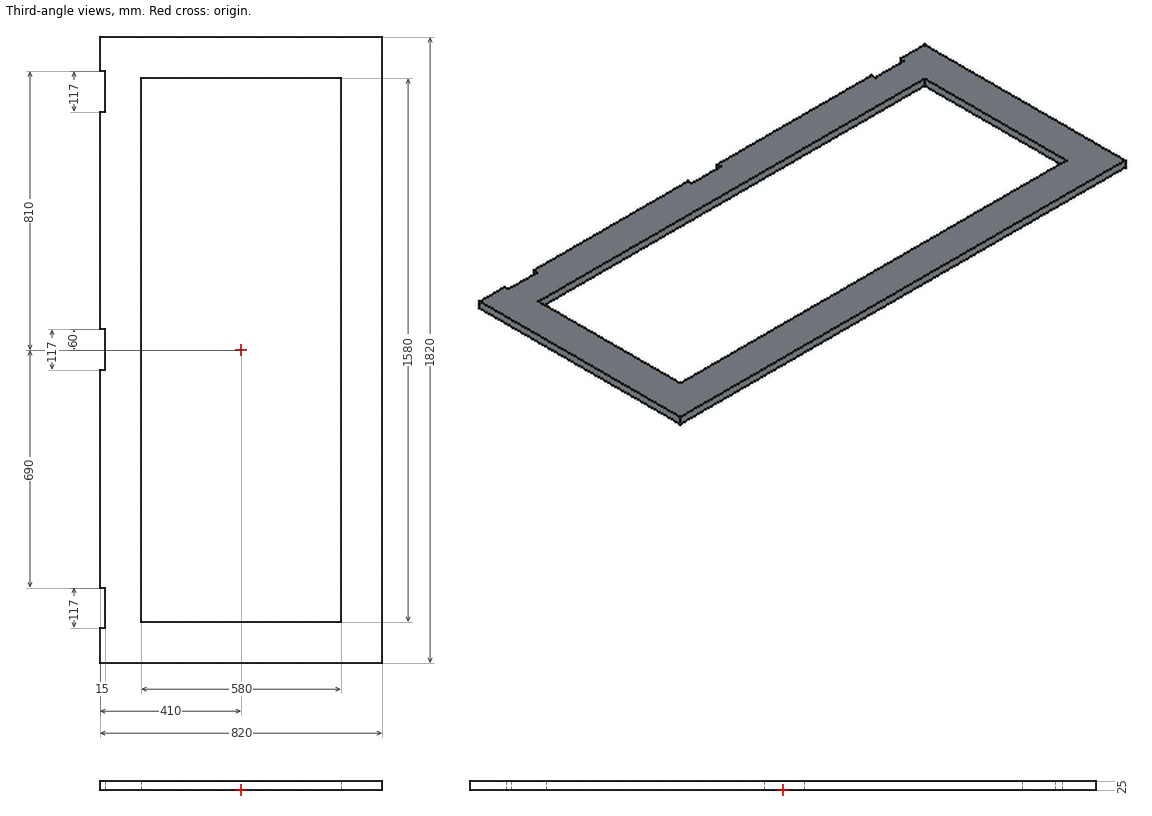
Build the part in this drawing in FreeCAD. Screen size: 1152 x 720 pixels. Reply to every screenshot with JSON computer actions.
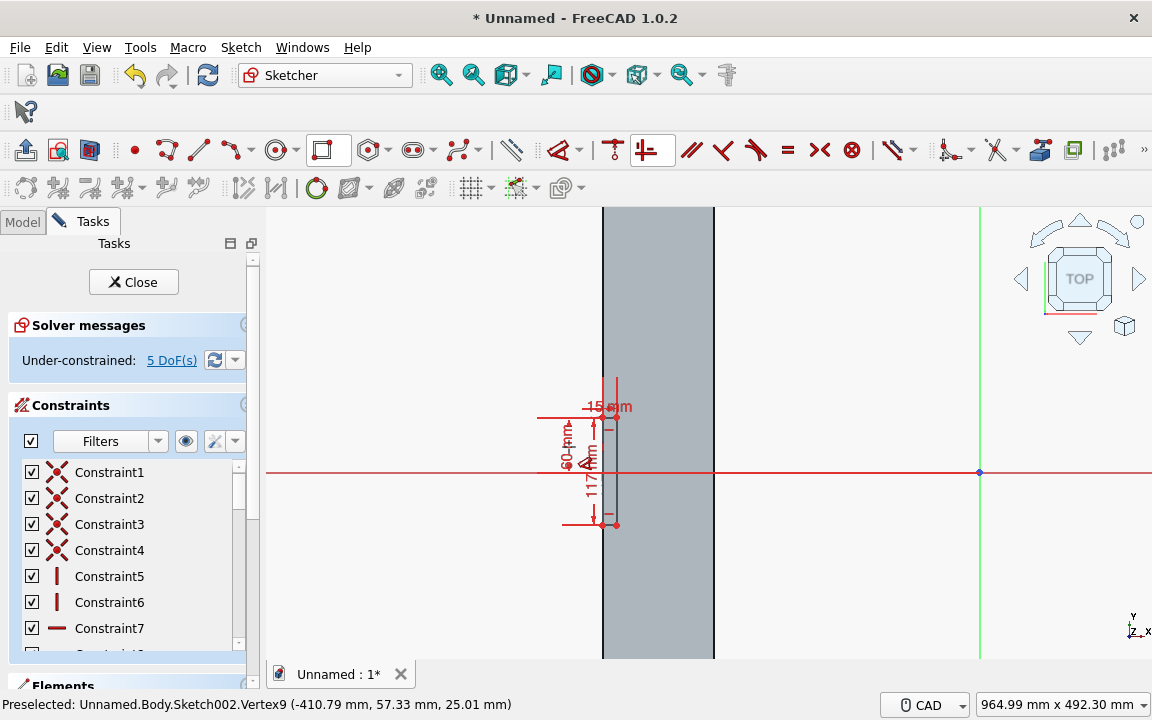
{"action": "scroll", "coordinate": [602, 423], "scroll_direction": "down", "scroll_amount": 8}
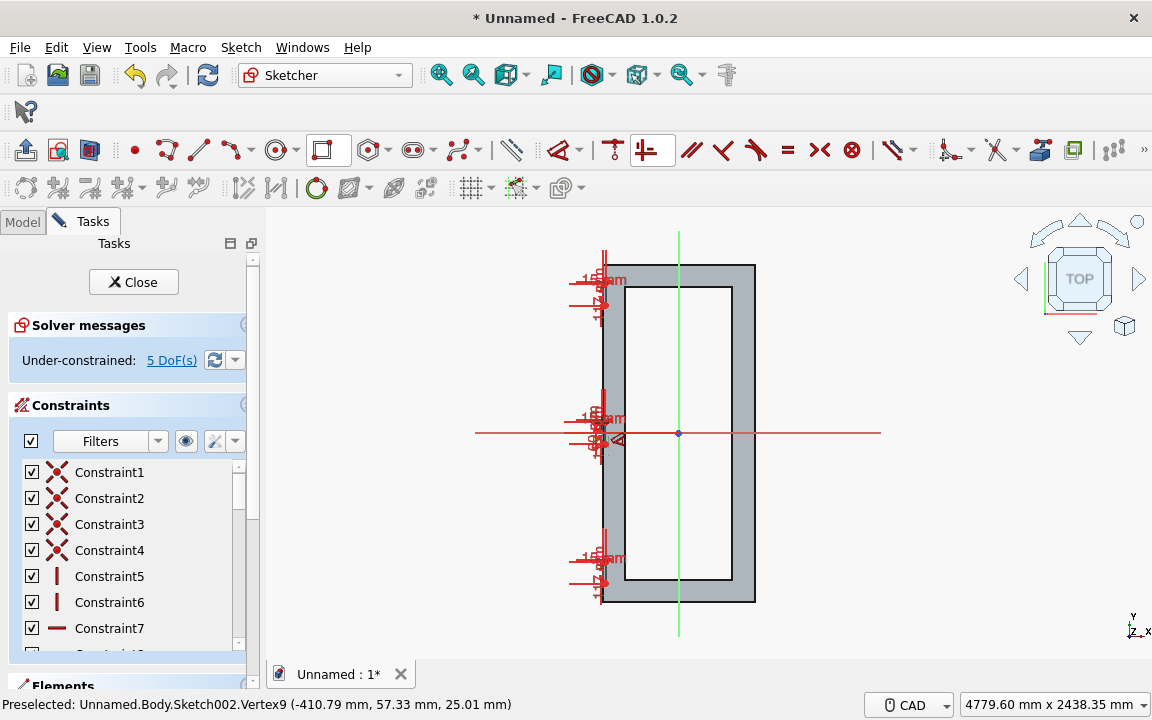
{"action": "scroll", "coordinate": [603, 562], "scroll_direction": "up", "scroll_amount": 8}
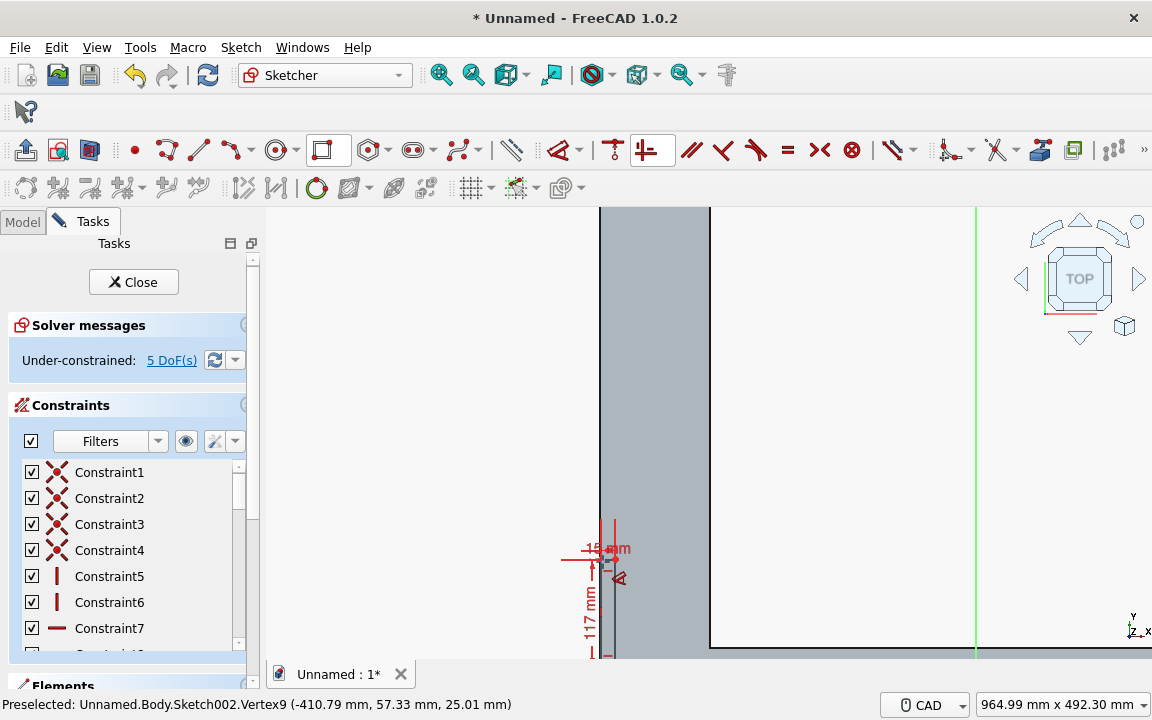
{"action": "left_click", "coordinate": [601, 560]}
{"action": "left_click", "coordinate": [789, 594]}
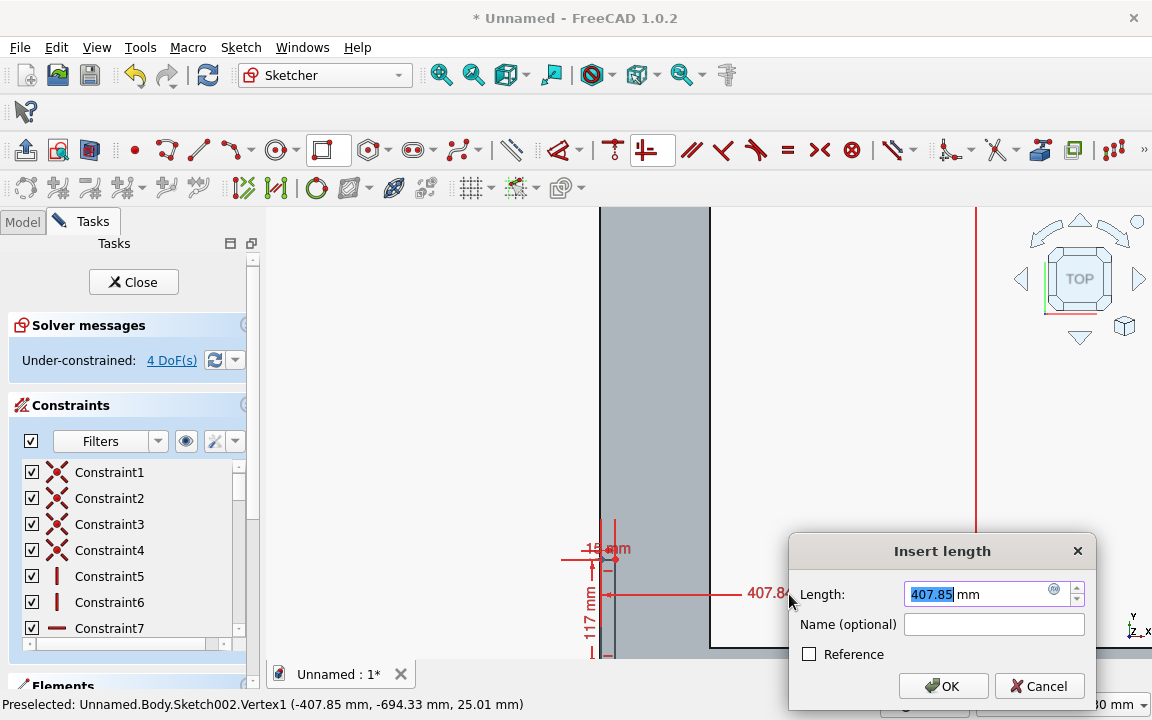
{"action": "type", "text": "410"}
{"action": "key", "text": "Return"}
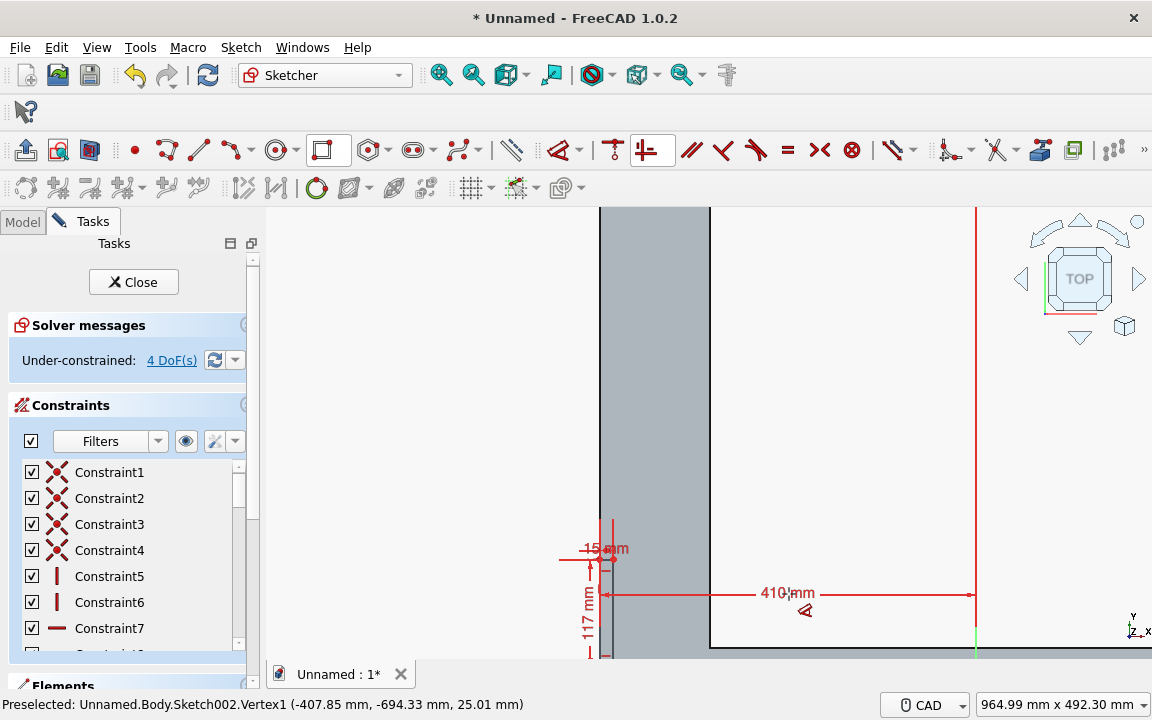
{"action": "left_click", "coordinate": [600, 560]}
{"action": "left_click", "coordinate": [566, 397]}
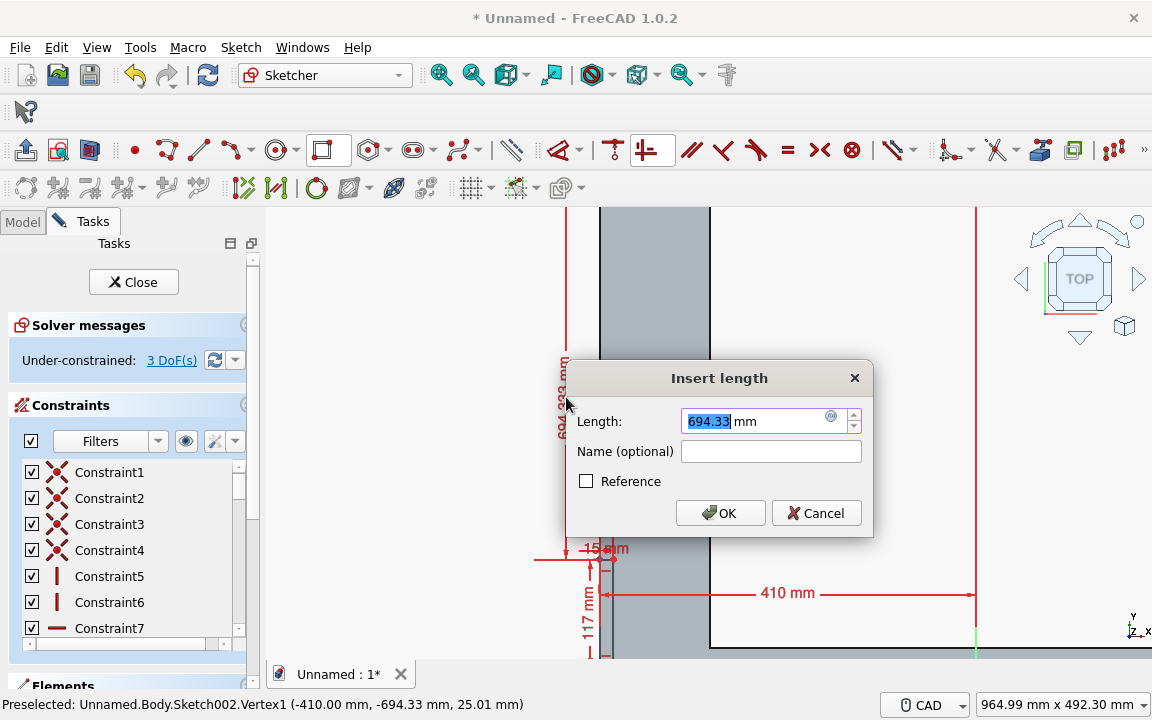
{"action": "type", "text": "690"}
{"action": "key", "text": "Return"}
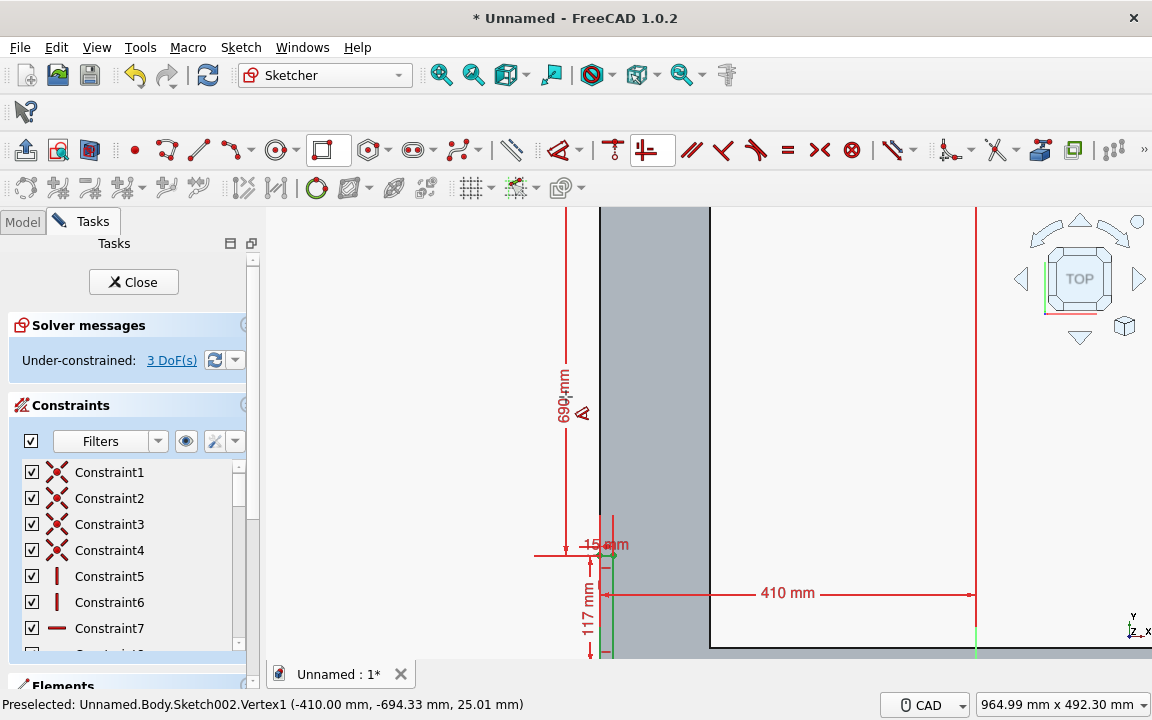
{"action": "scroll", "coordinate": [603, 563], "scroll_direction": "down", "scroll_amount": 8}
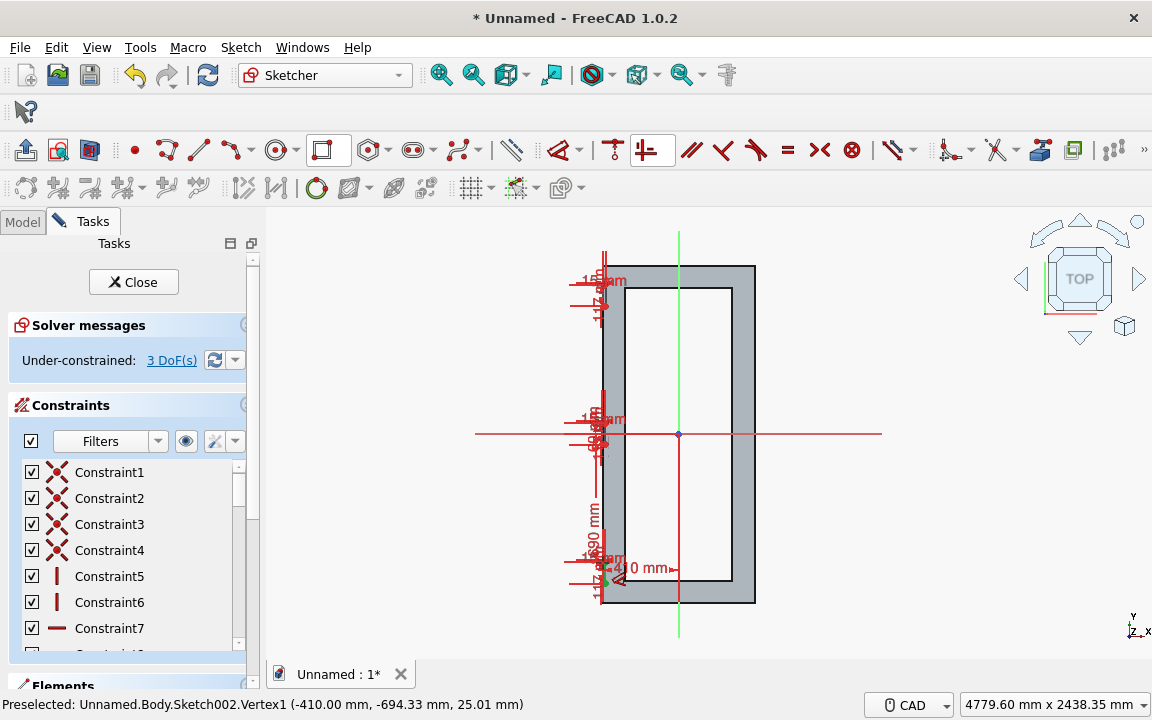
{"action": "scroll", "coordinate": [602, 423], "scroll_direction": "up", "scroll_amount": 8}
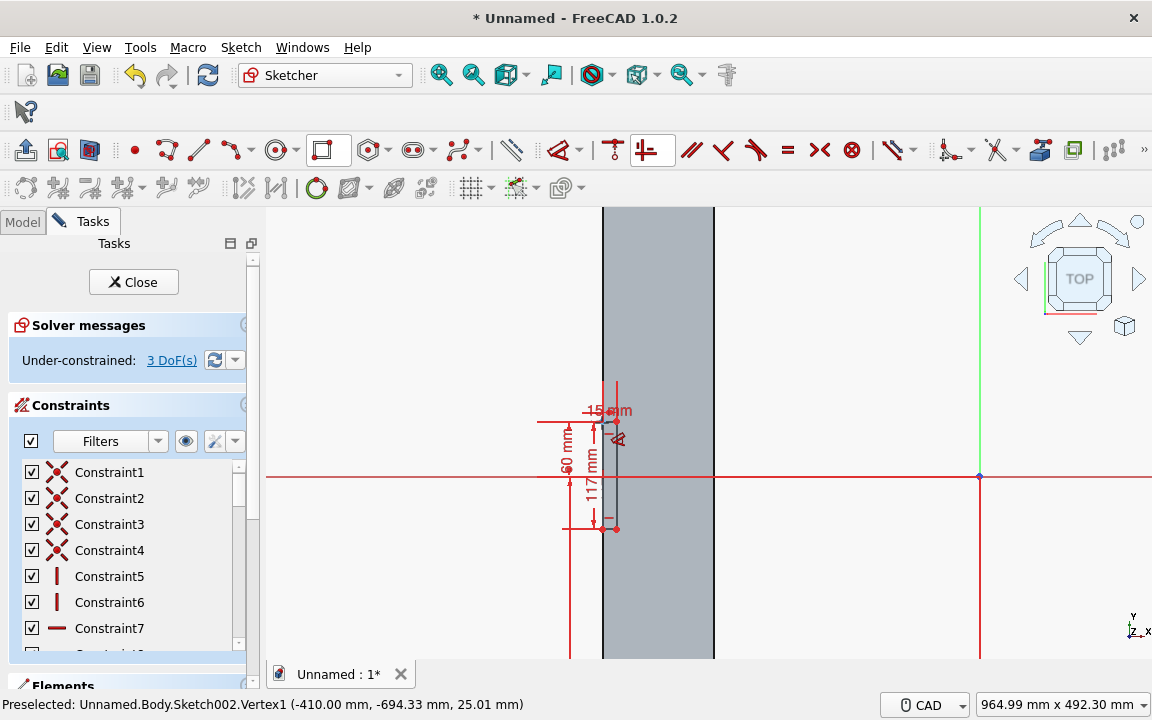
{"action": "left_click", "coordinate": [603, 422]}
{"action": "left_click", "coordinate": [791, 388]}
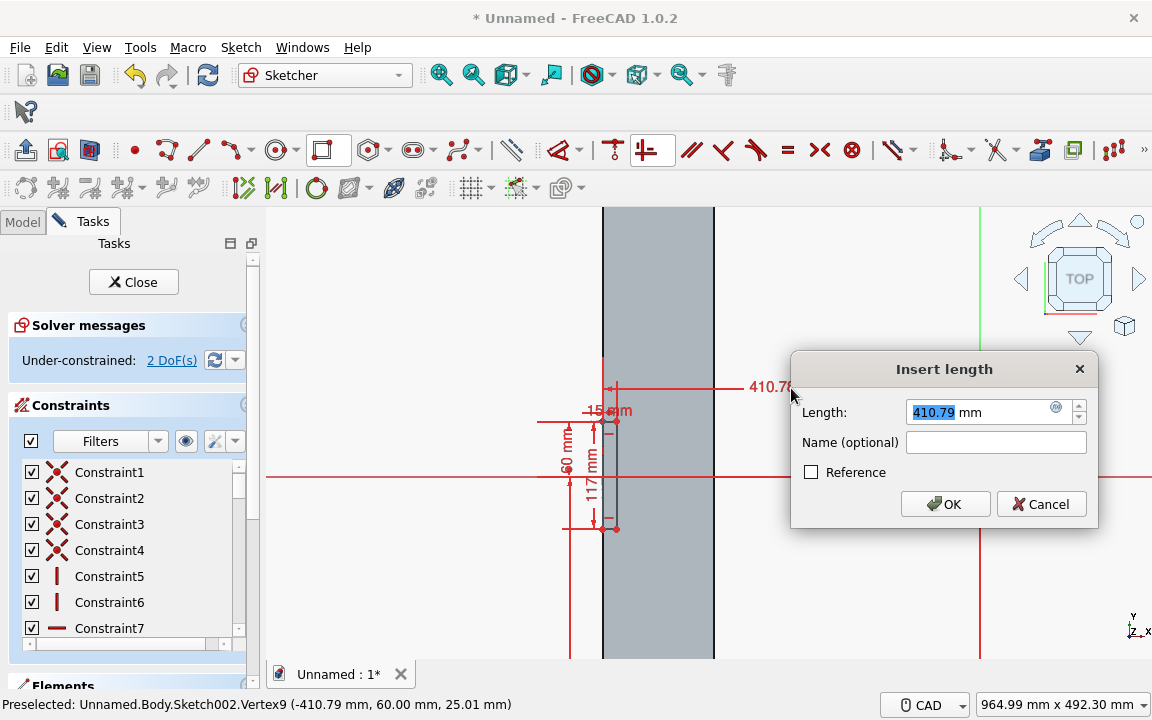
{"action": "type", "text": "410"}
{"action": "key", "text": "Return"}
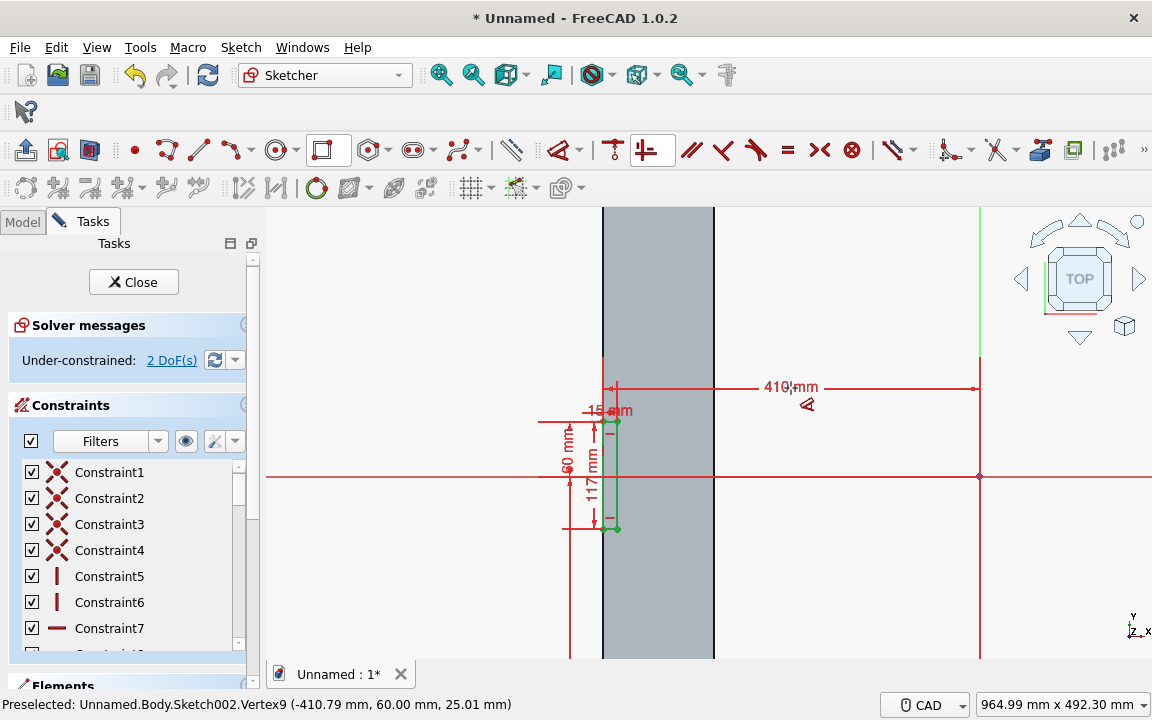
{"action": "scroll", "coordinate": [602, 422], "scroll_direction": "down", "scroll_amount": 8}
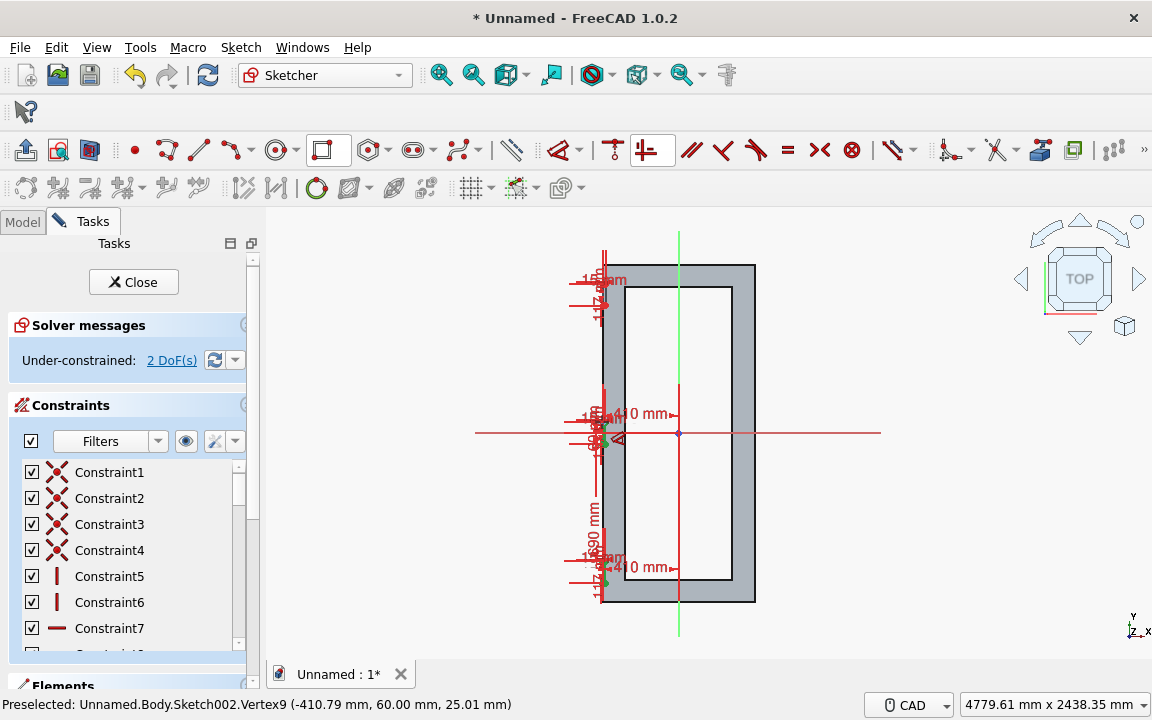
{"action": "scroll", "coordinate": [603, 284], "scroll_direction": "up", "scroll_amount": 8}